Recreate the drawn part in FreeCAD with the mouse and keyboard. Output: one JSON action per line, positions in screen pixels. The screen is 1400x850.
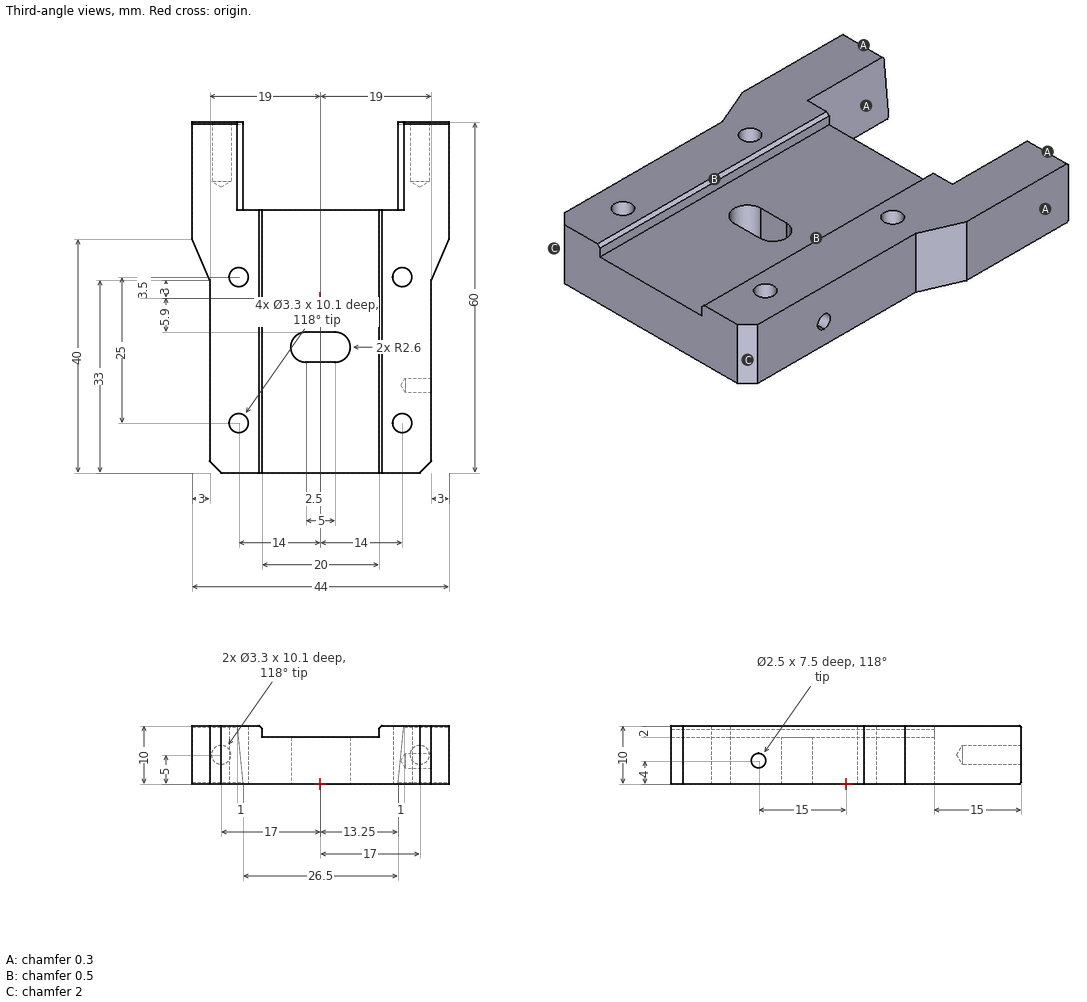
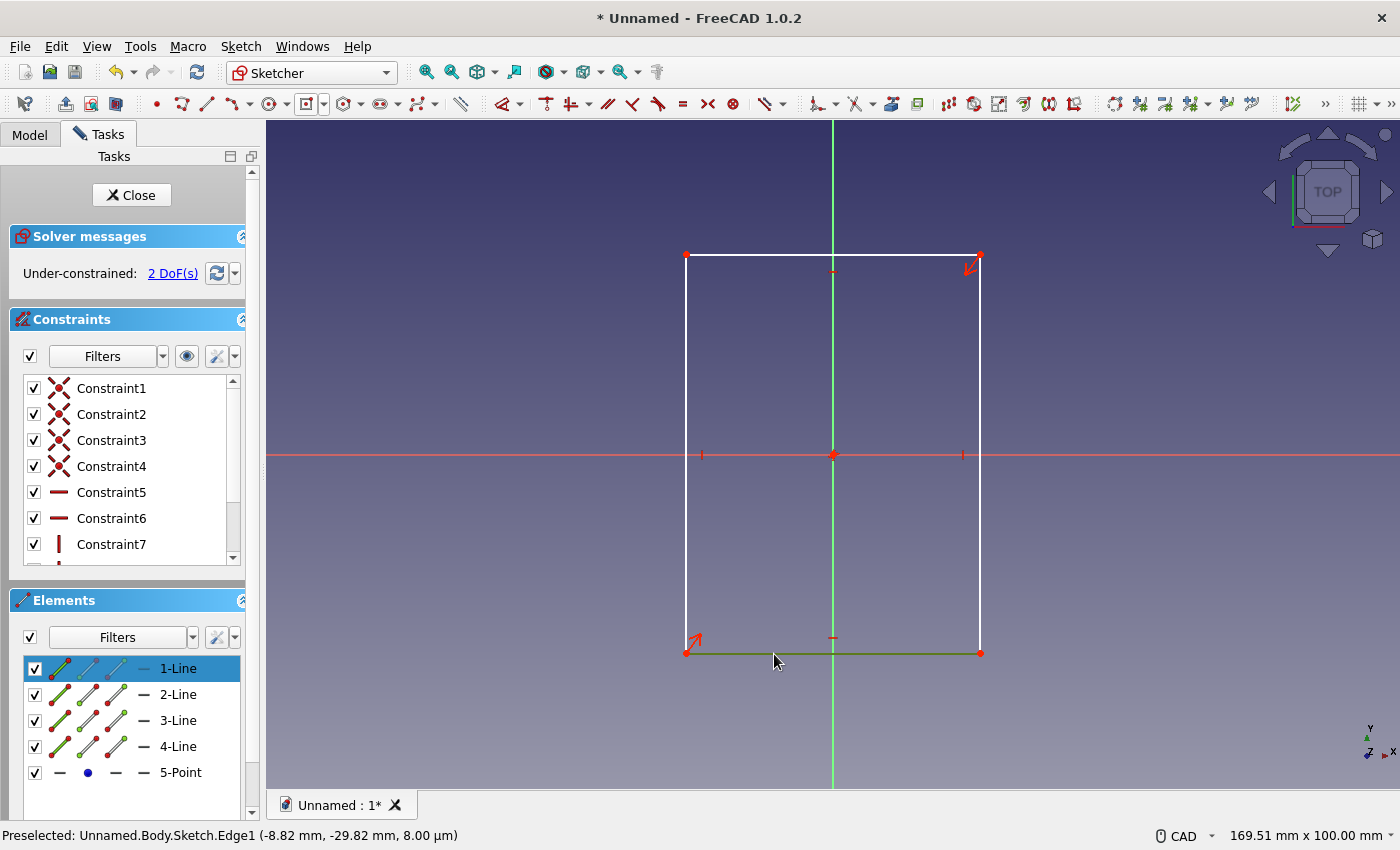
{"action": "key", "text": "l"}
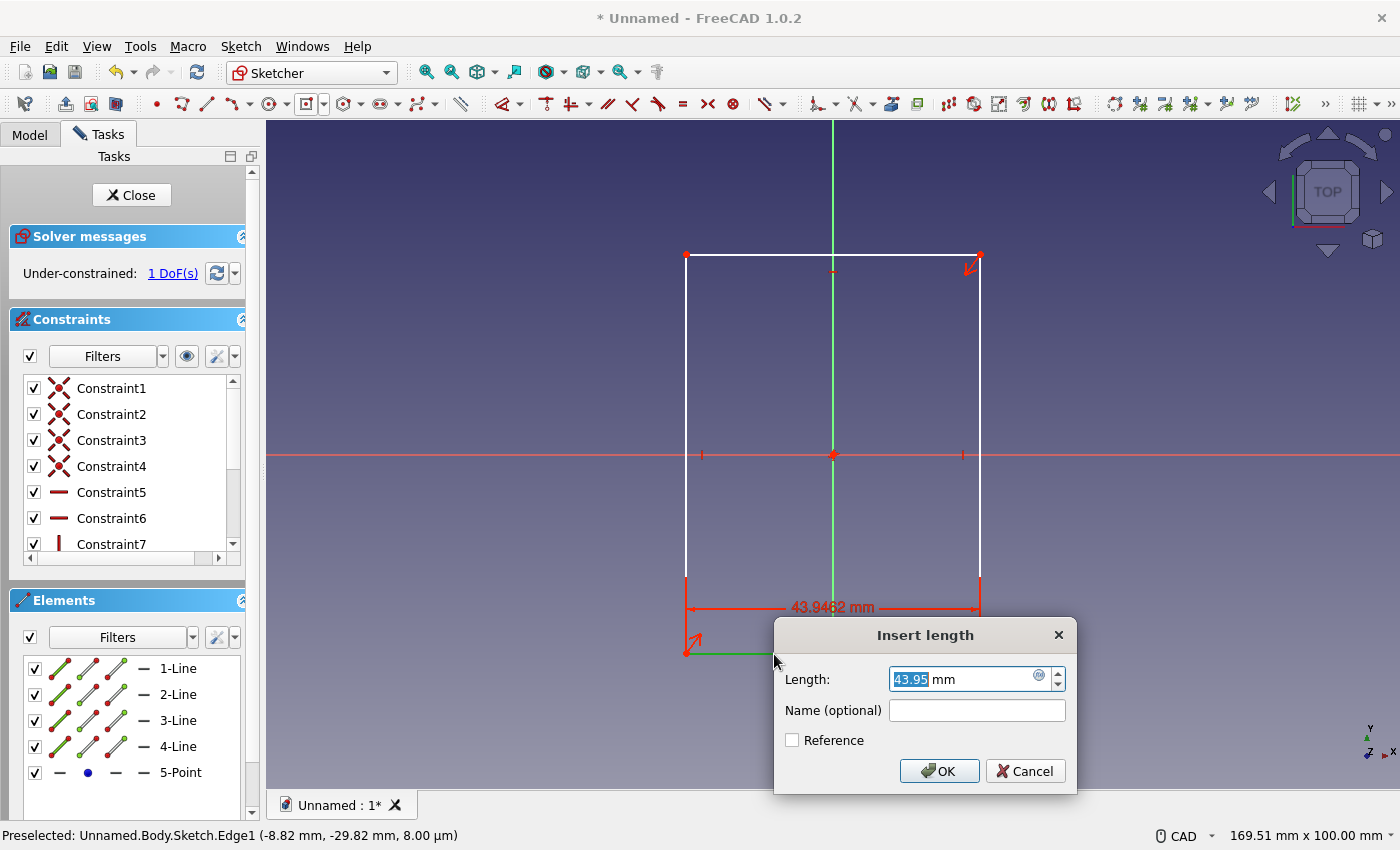
{"action": "type", "text": "44"}
{"action": "key", "text": "Return"}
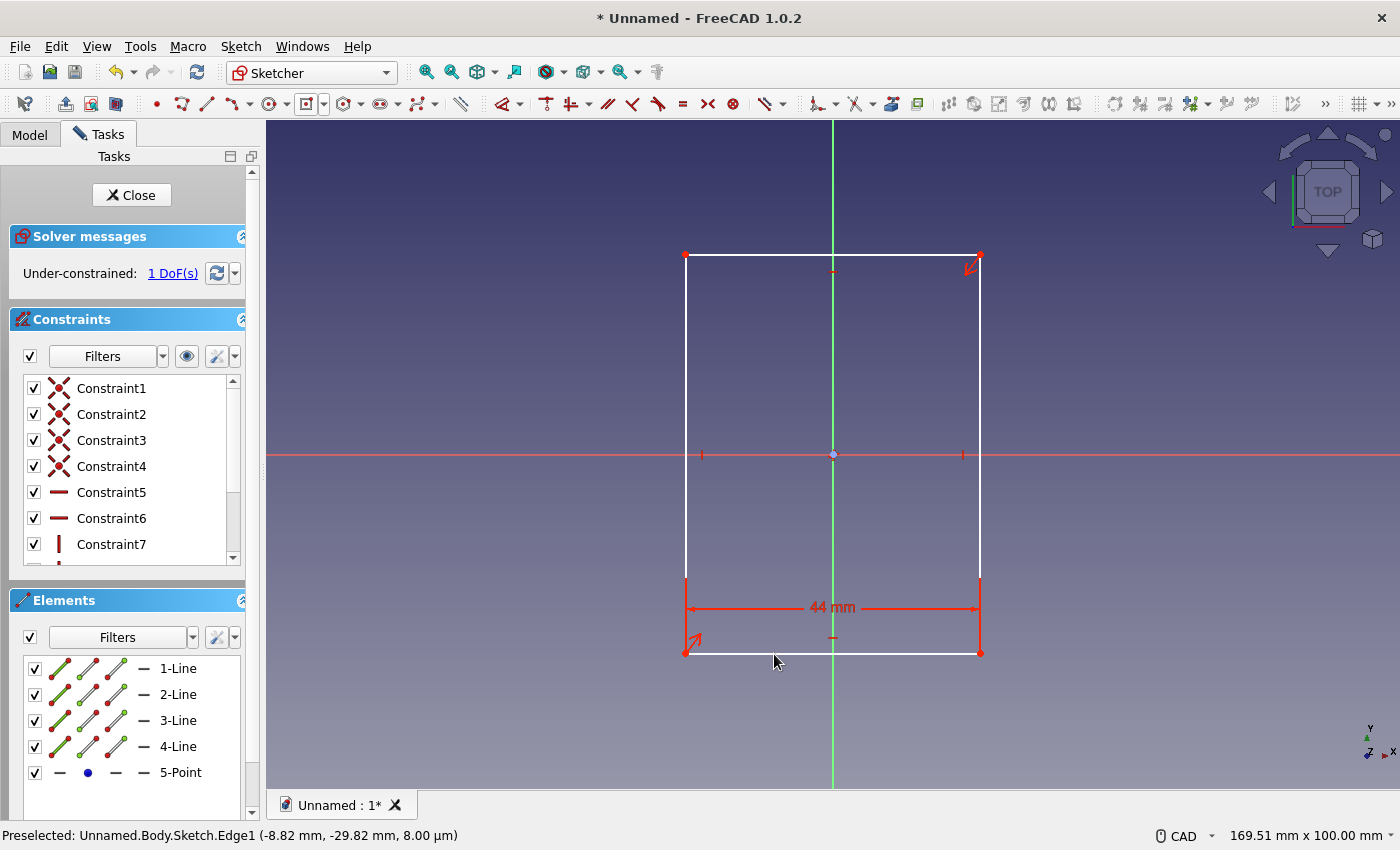
{"action": "left_click", "coordinate": [980, 534]}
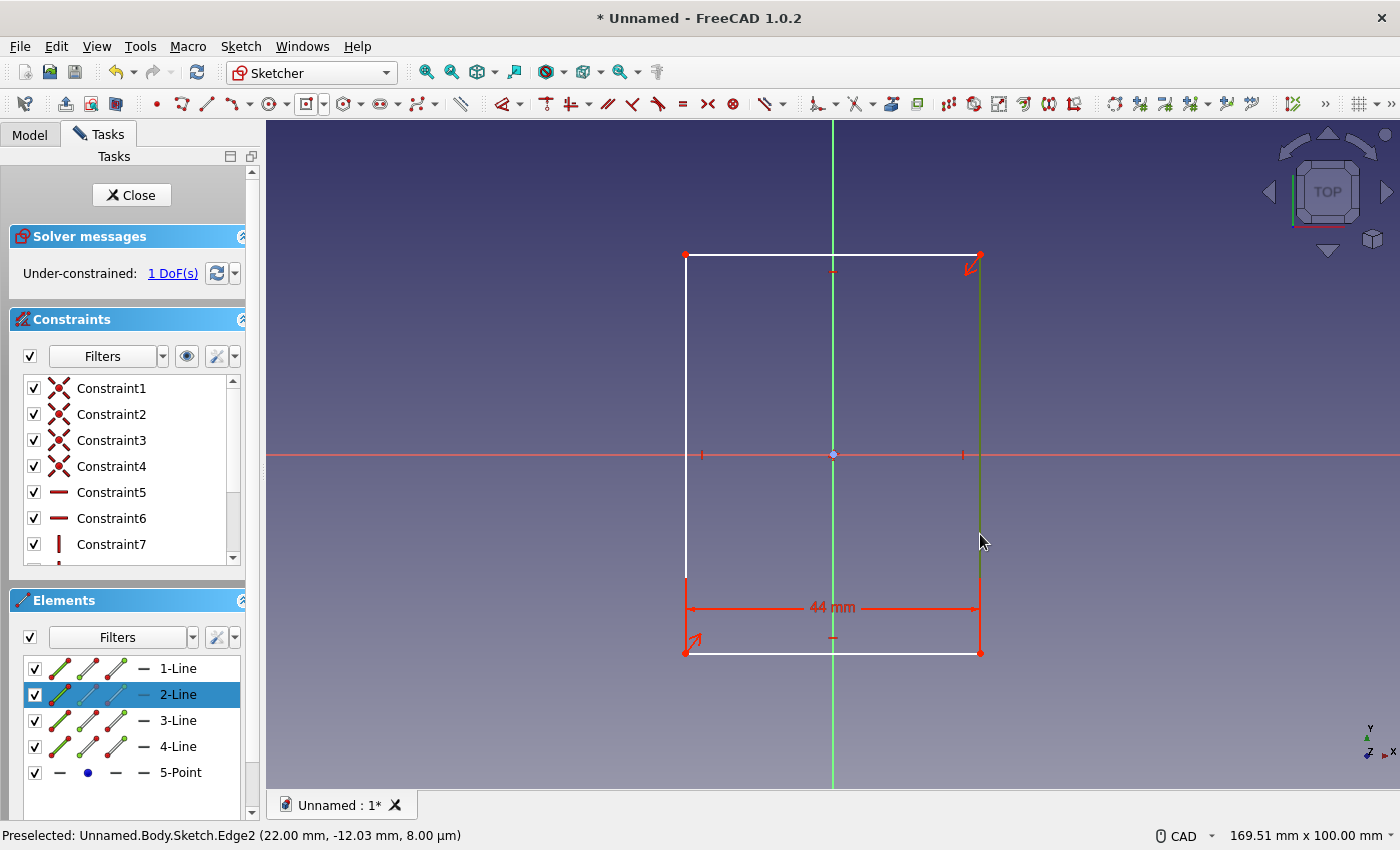
{"action": "left_click", "coordinate": [520, 104]}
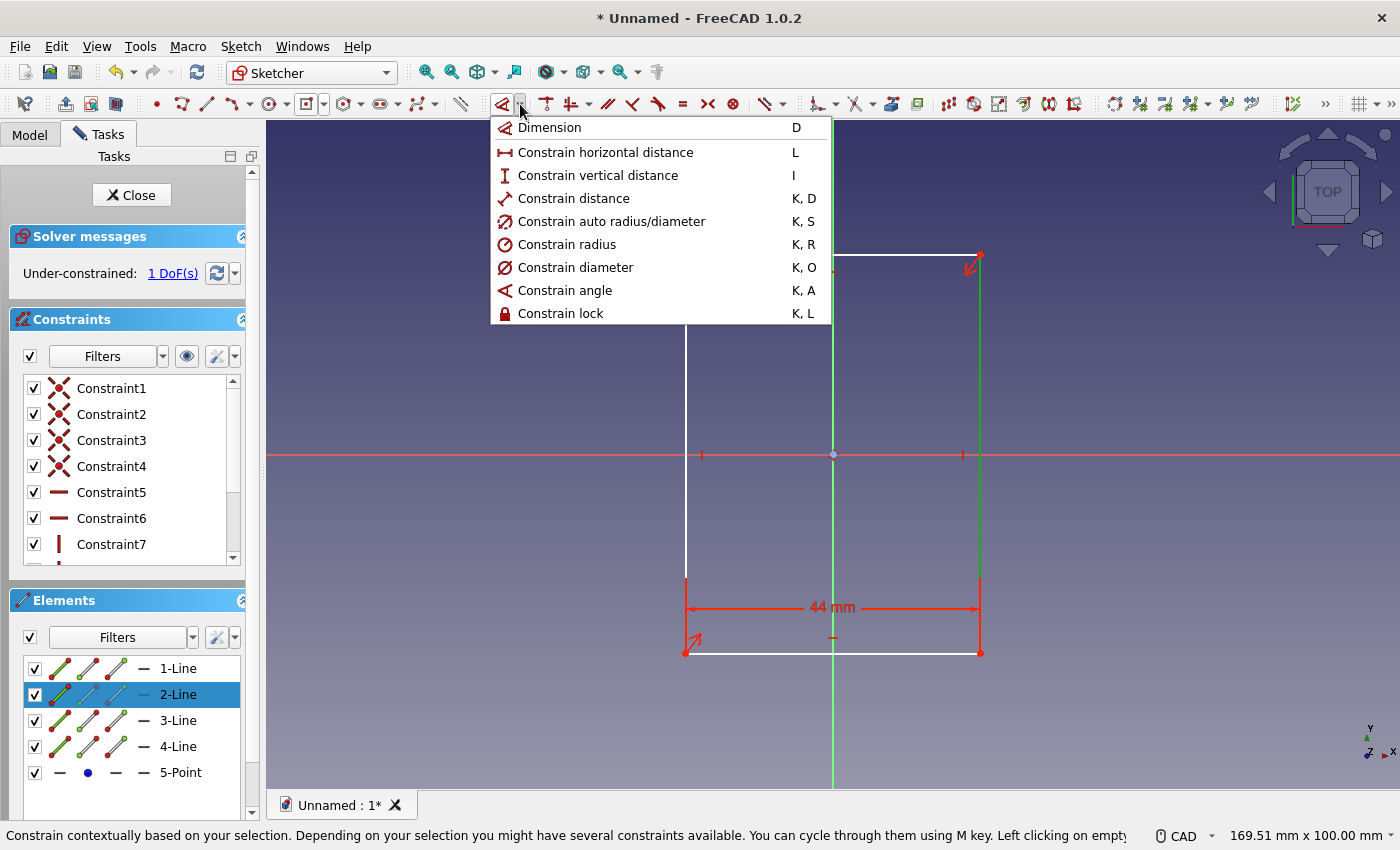
{"action": "left_click", "coordinate": [661, 176]}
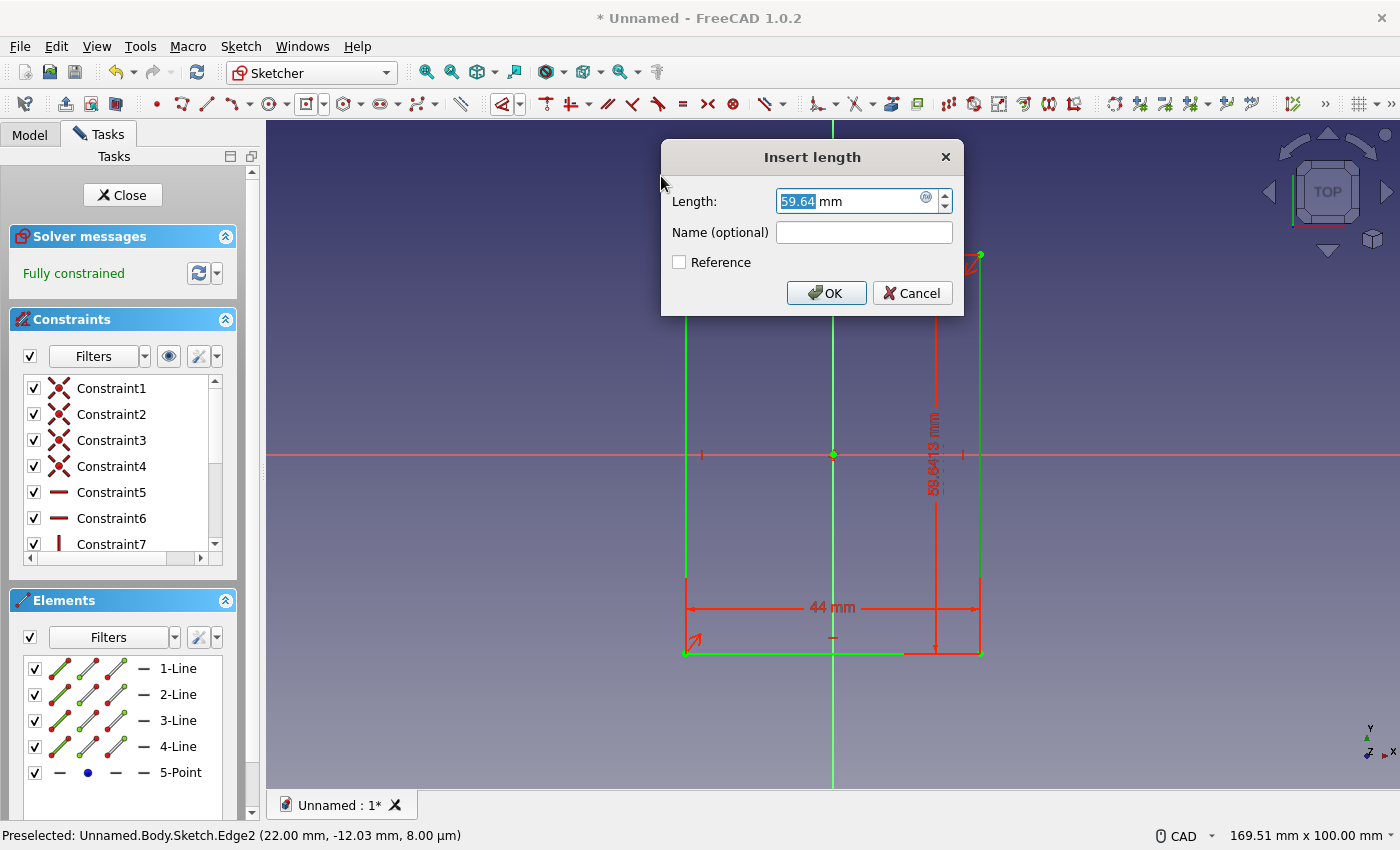
{"action": "type", "text": "60"}
{"action": "key", "text": "Return"}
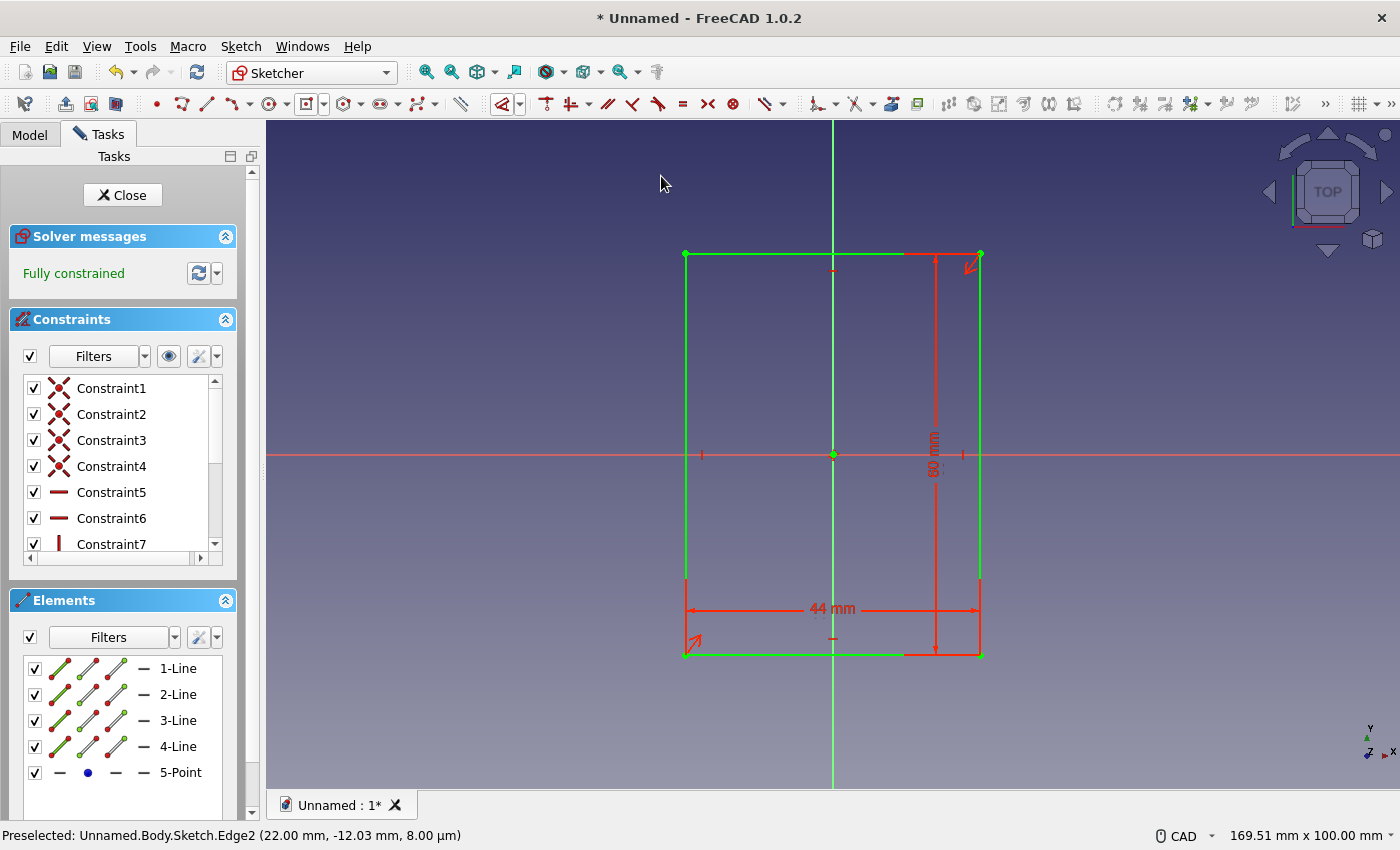
{"action": "left_click", "coordinate": [123, 195]}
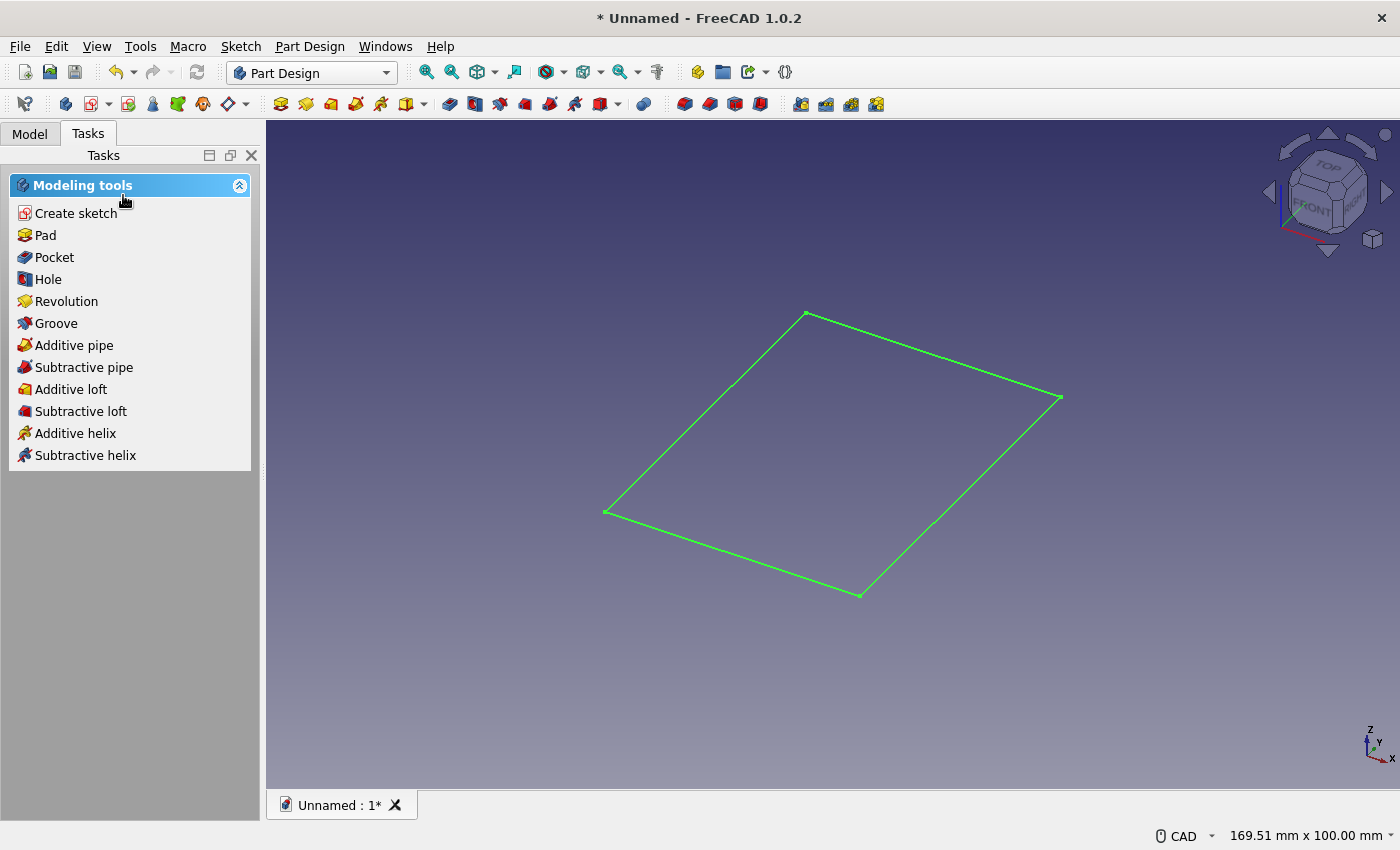
{"action": "left_click", "coordinate": [281, 104]}